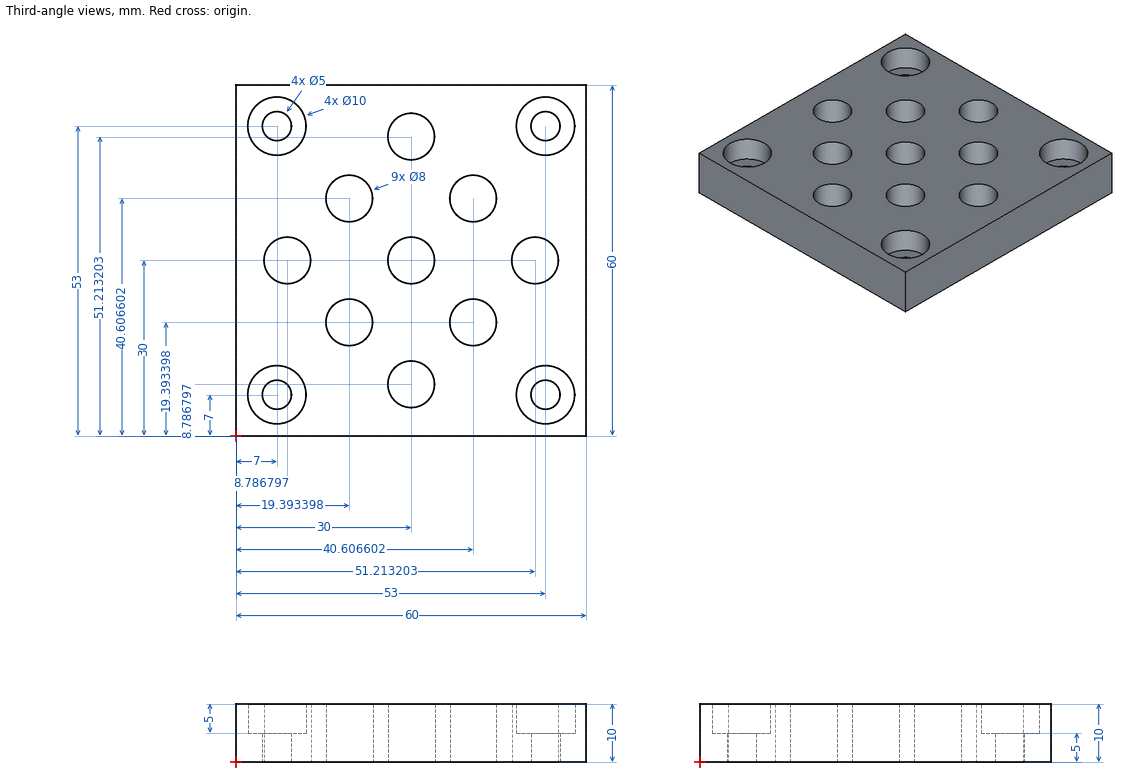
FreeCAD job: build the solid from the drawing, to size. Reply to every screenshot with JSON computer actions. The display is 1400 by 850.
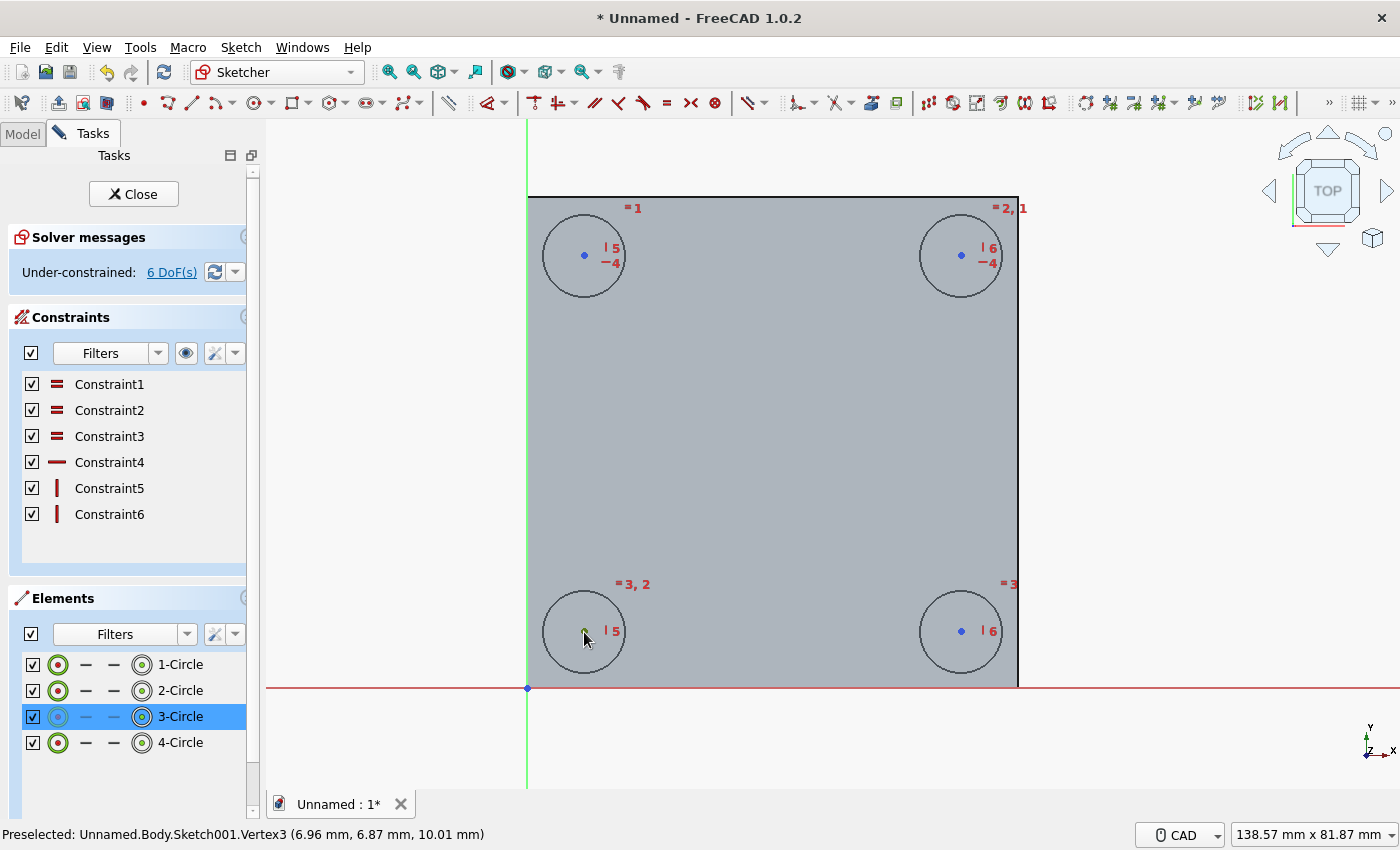
{"action": "left_click", "coordinate": [961, 632]}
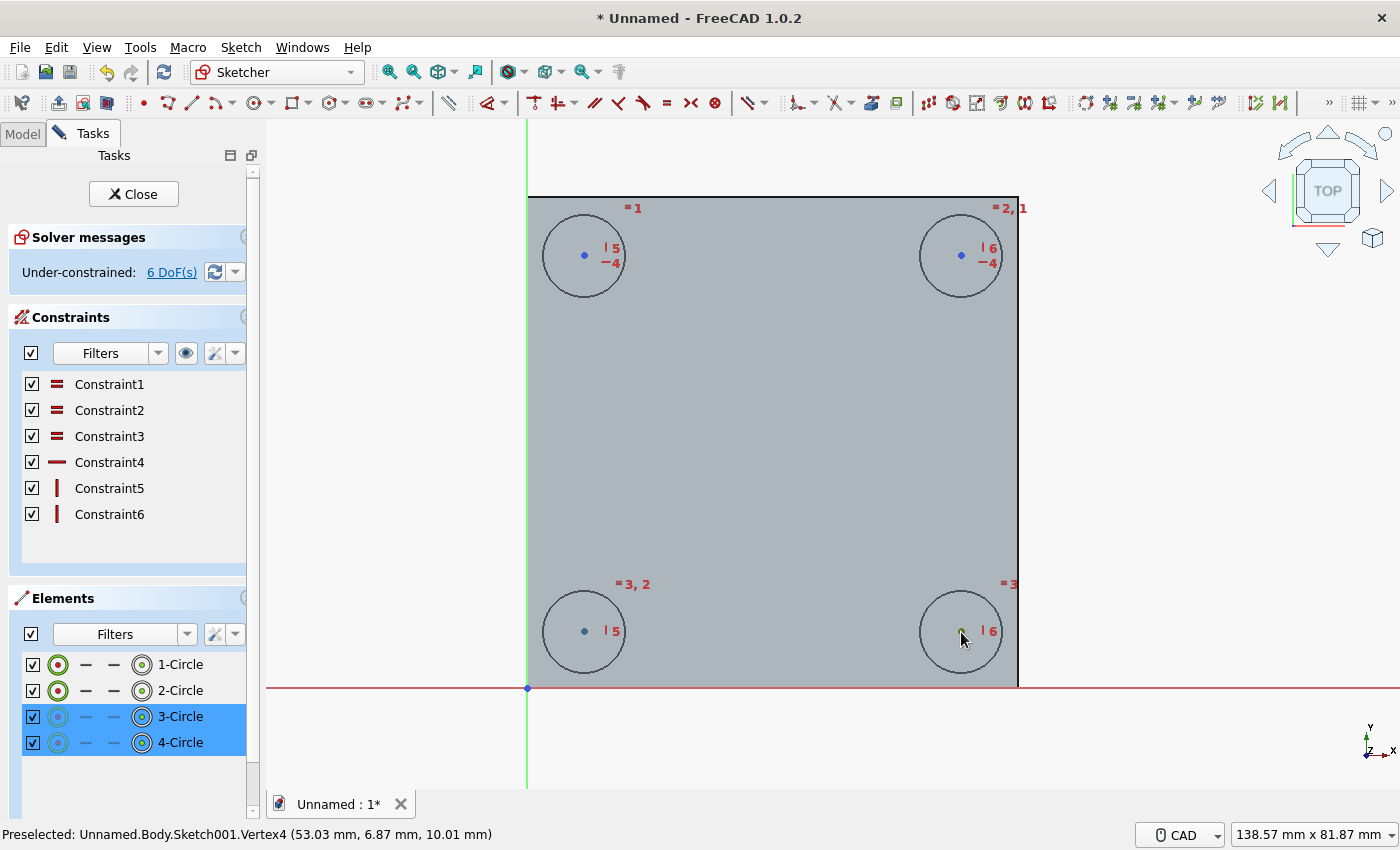
{"action": "left_click", "coordinate": [576, 104]}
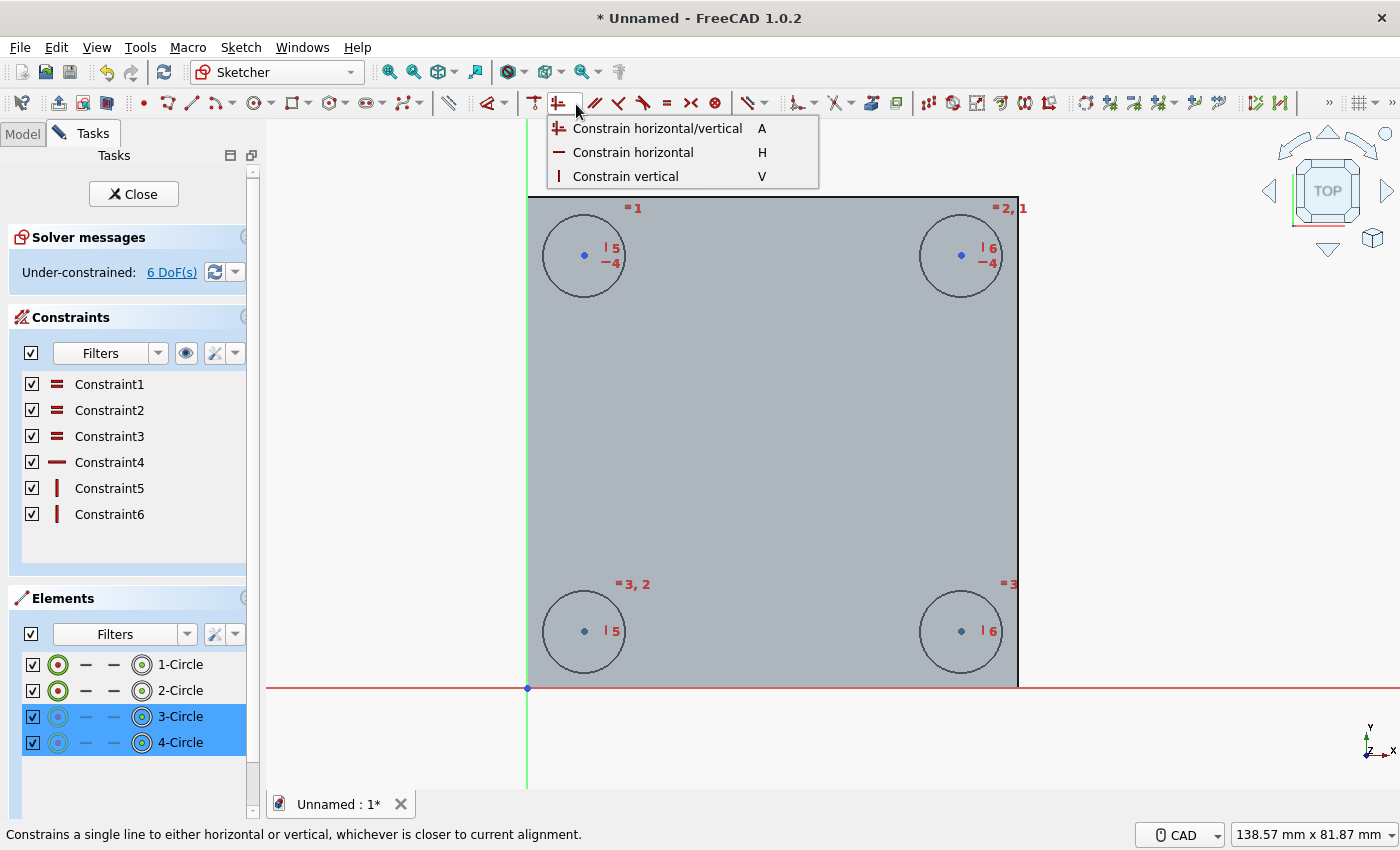
{"action": "left_click", "coordinate": [683, 152]}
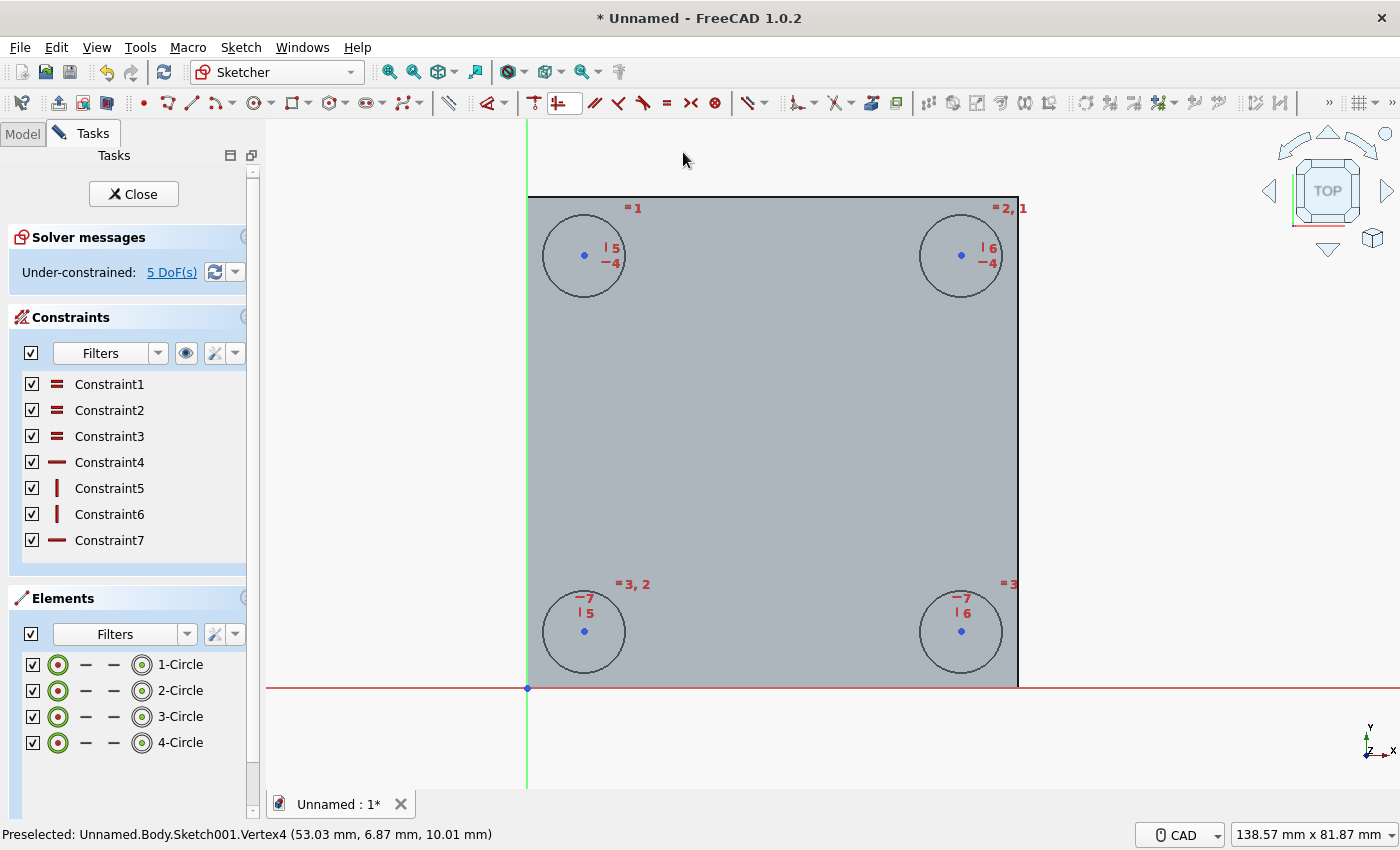
{"action": "left_click", "coordinate": [488, 104]}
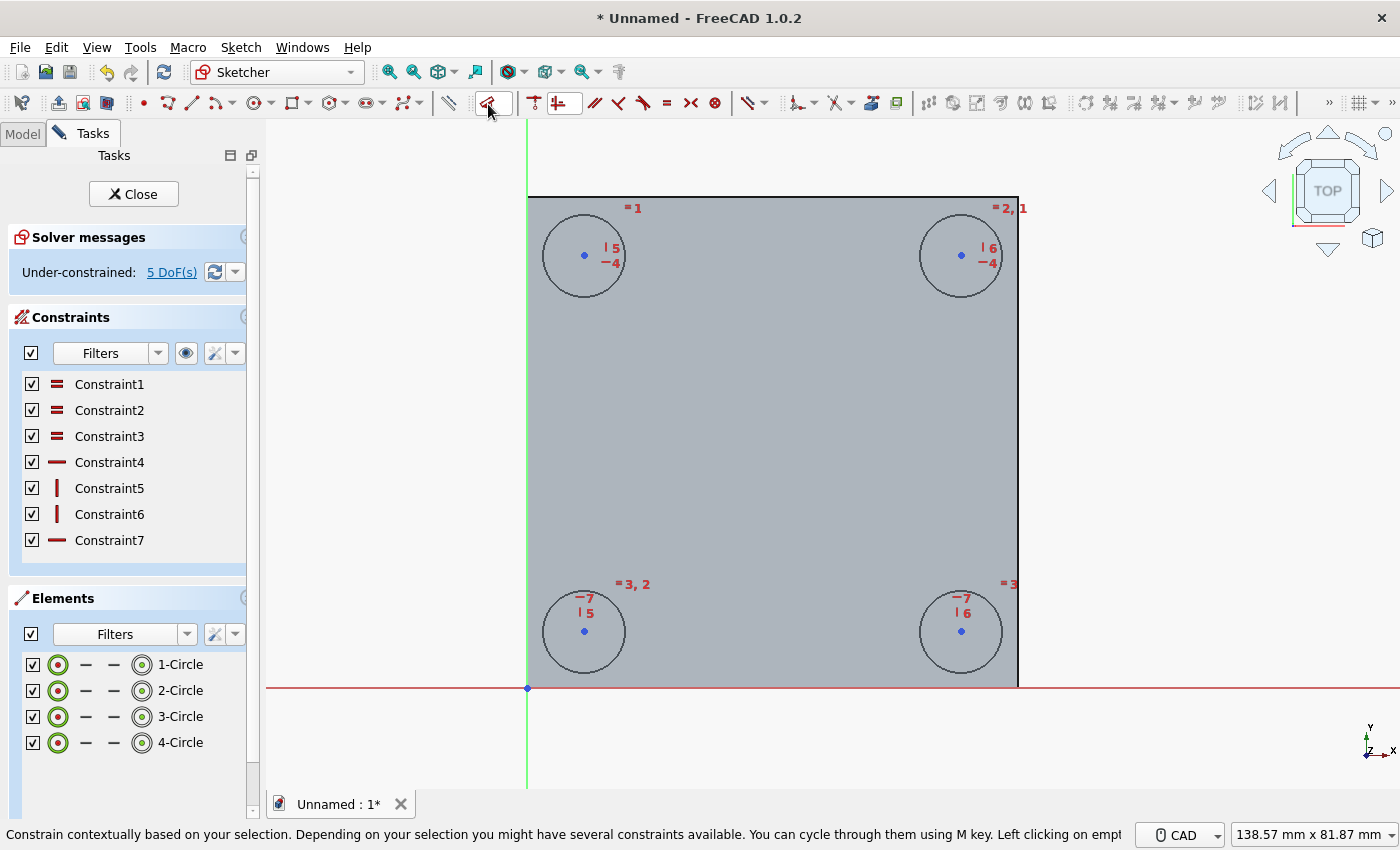
{"action": "left_click", "coordinate": [613, 227]}
{"action": "left_click", "coordinate": [636, 204]}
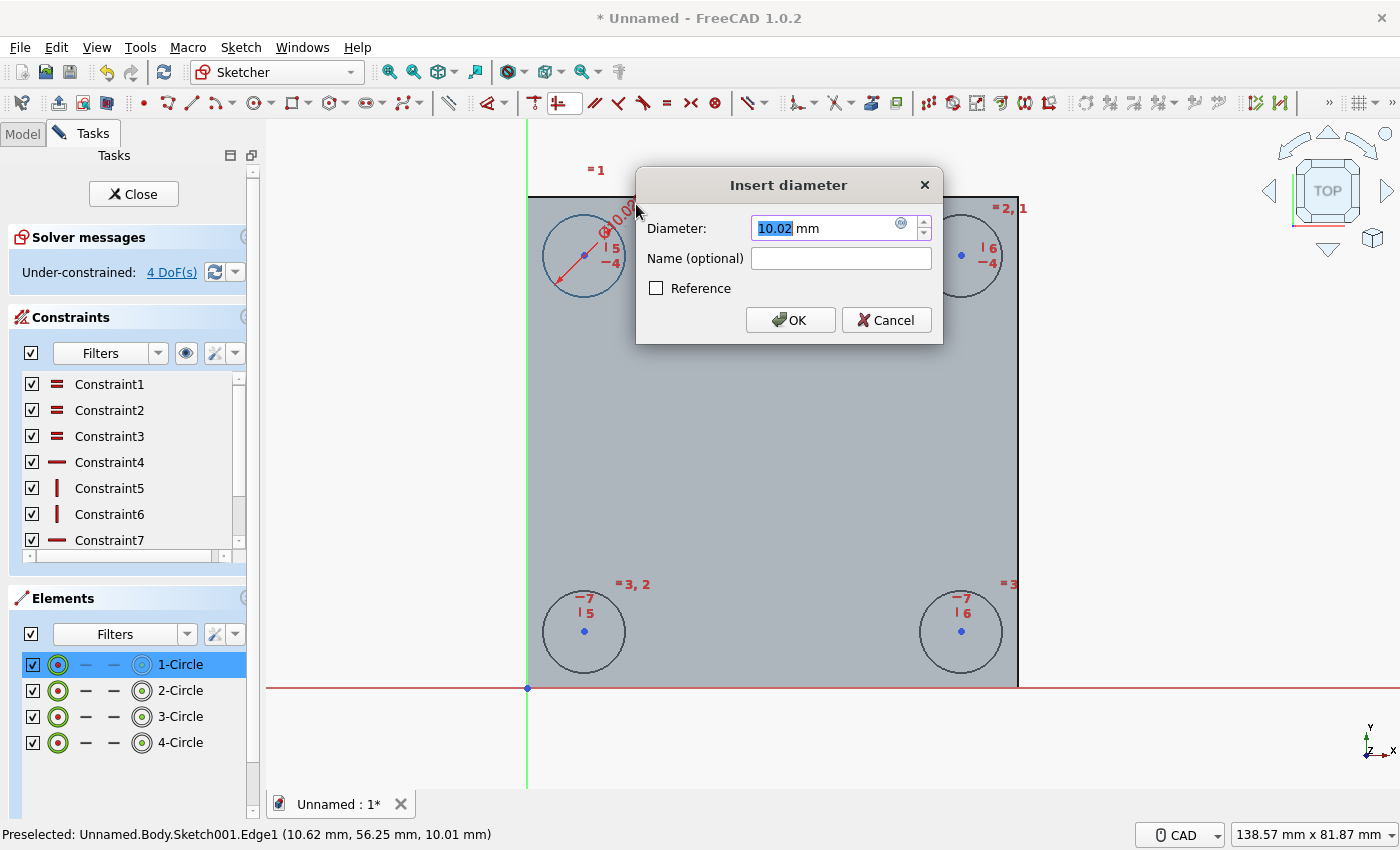
{"action": "type", "text": "10"}
{"action": "key", "text": "Return"}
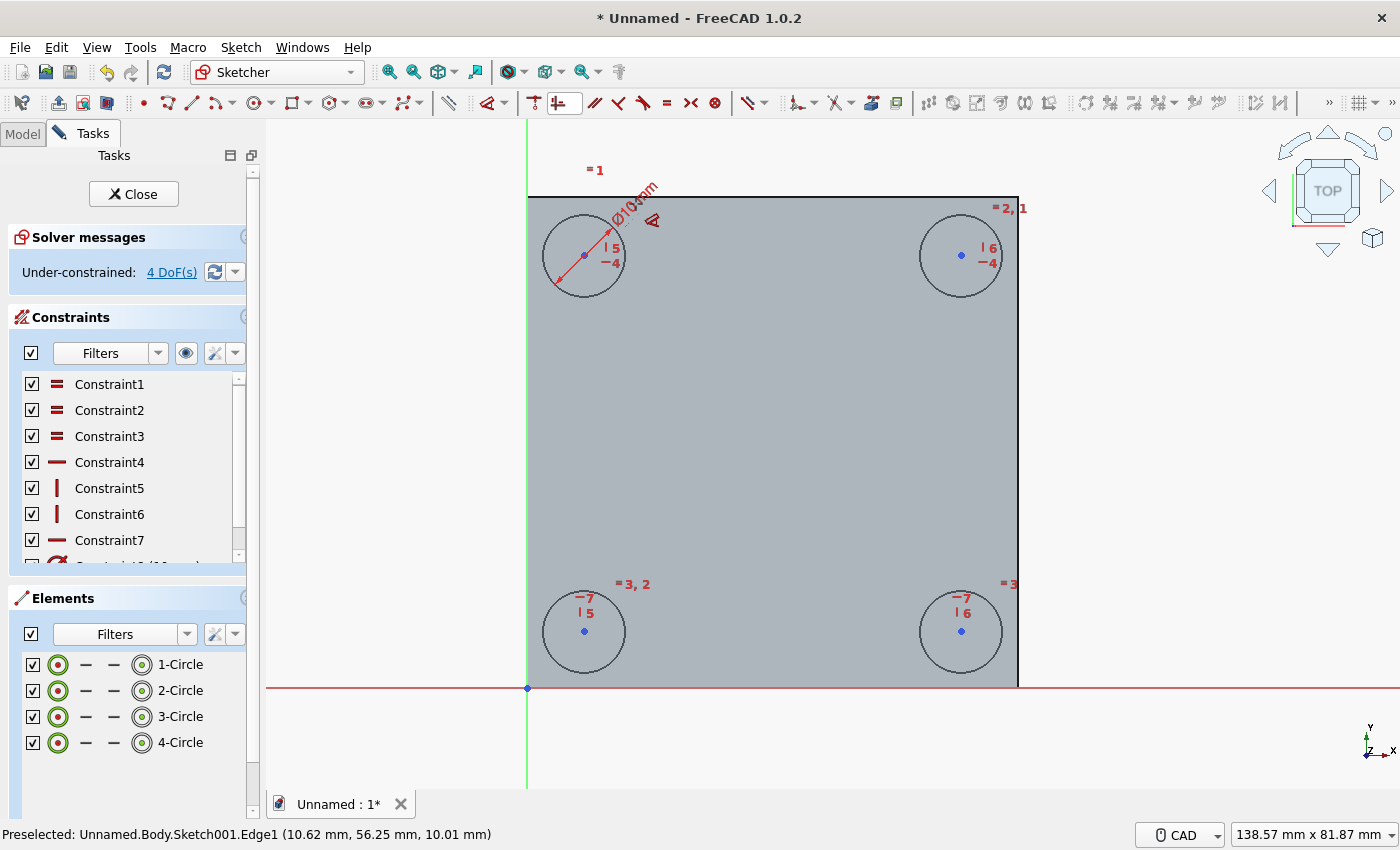
{"action": "left_click", "coordinate": [584, 256]}
{"action": "left_click", "coordinate": [556, 722]}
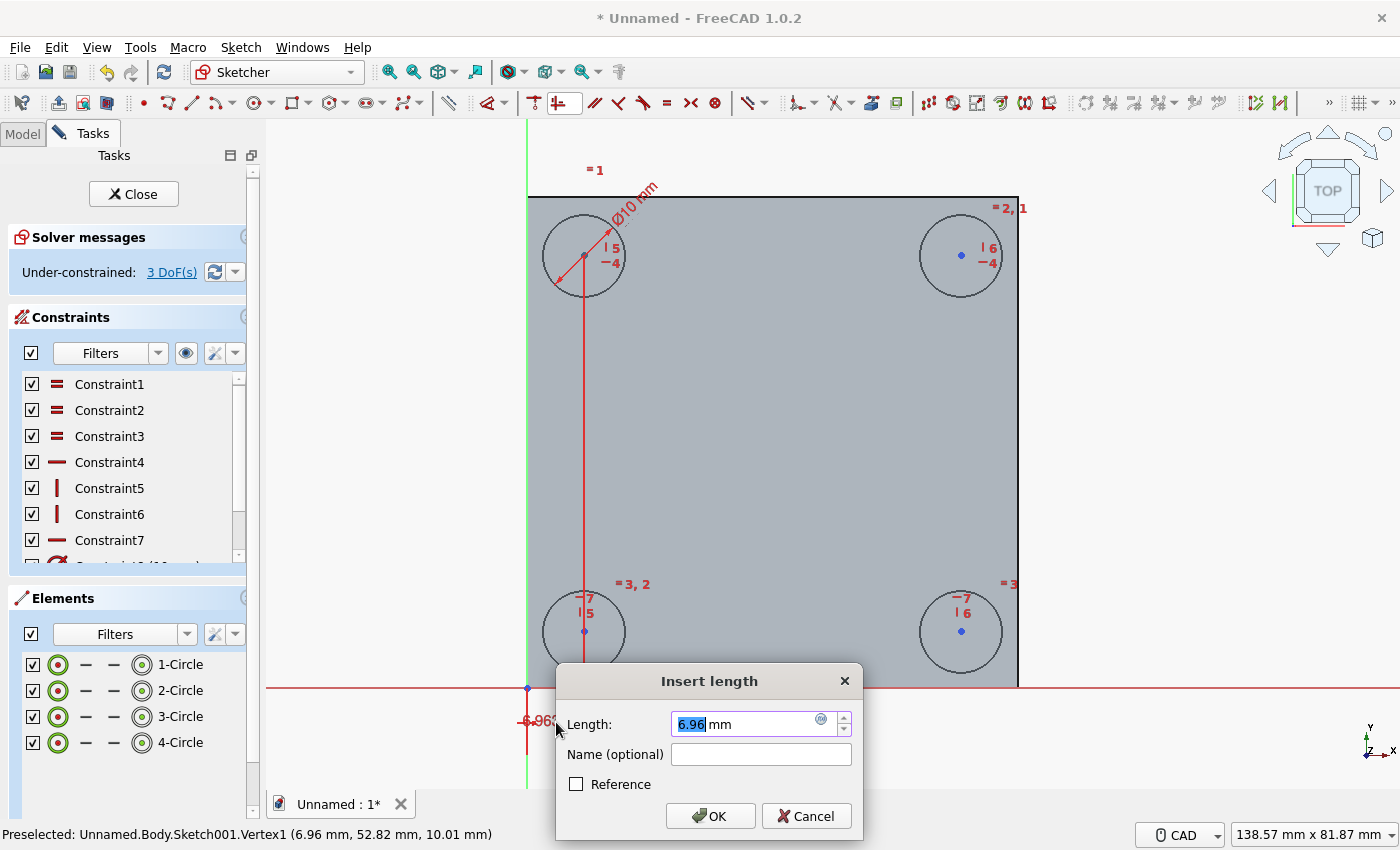
{"action": "type", "text": "7"}
{"action": "key", "text": "Return"}